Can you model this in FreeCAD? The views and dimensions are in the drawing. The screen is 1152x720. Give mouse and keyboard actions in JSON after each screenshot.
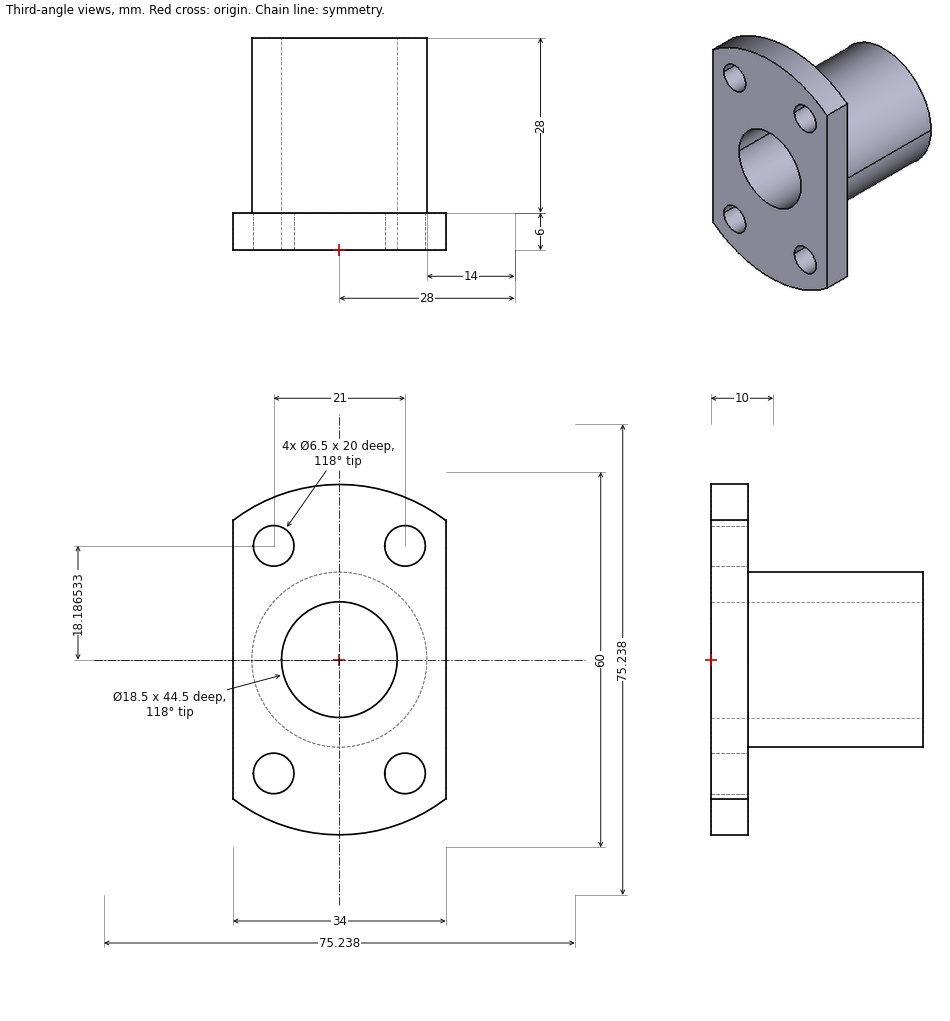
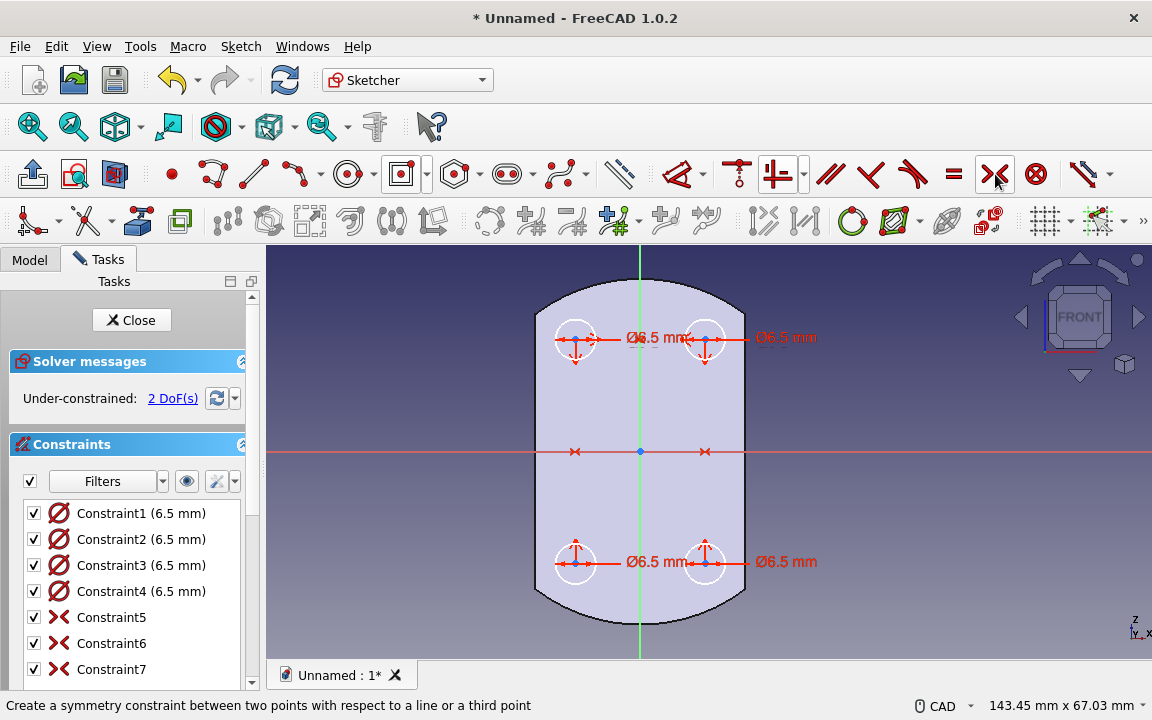
{"action": "left_click", "coordinate": [676, 174]}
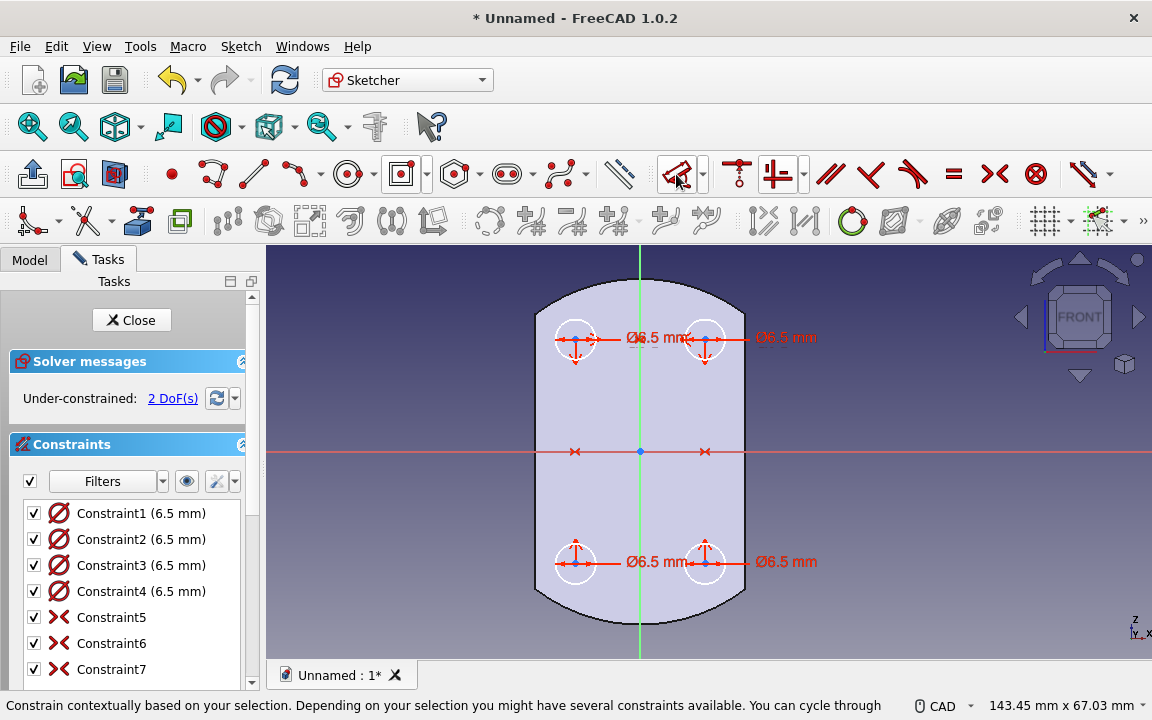
{"action": "left_click", "coordinate": [576, 340]}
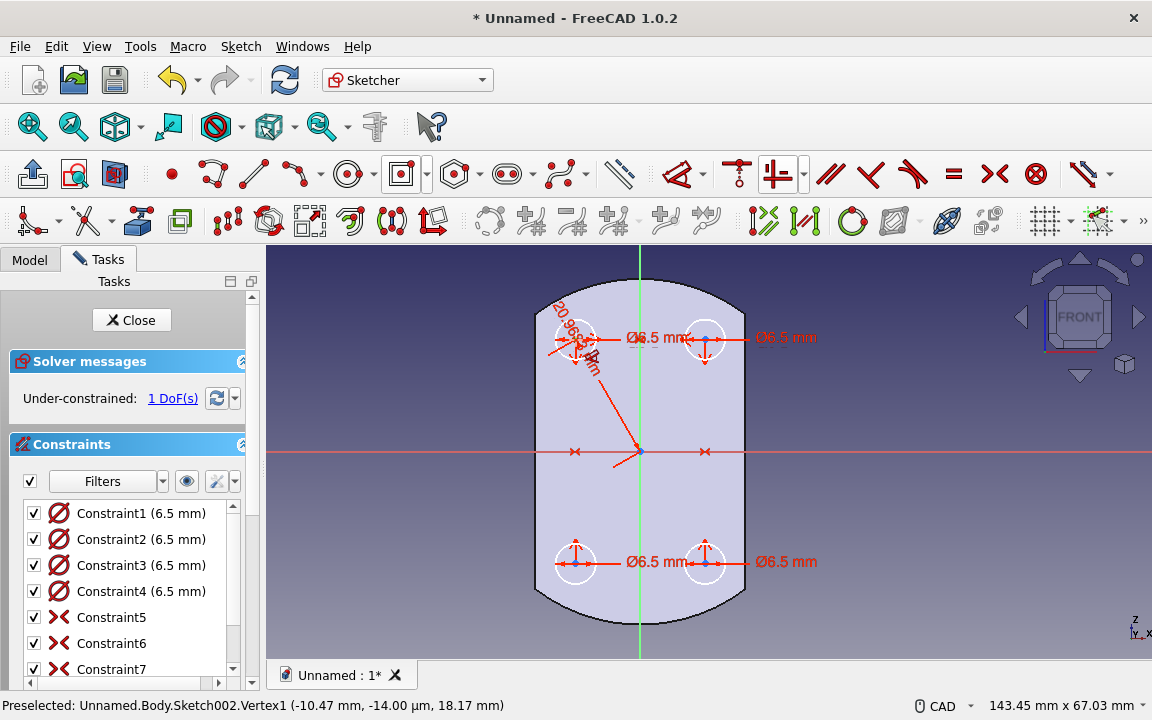
{"action": "left_click", "coordinate": [705, 340]}
{"action": "left_click", "coordinate": [611, 306]}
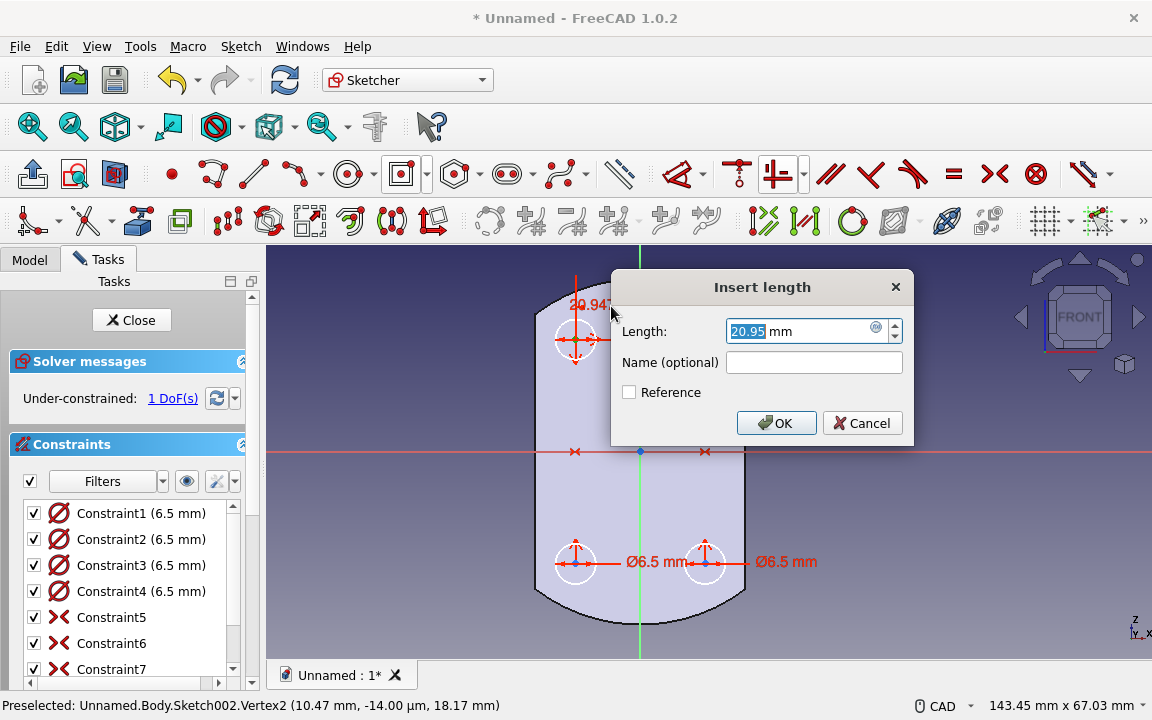
{"action": "type", "text": "21"}
{"action": "key", "text": "Return"}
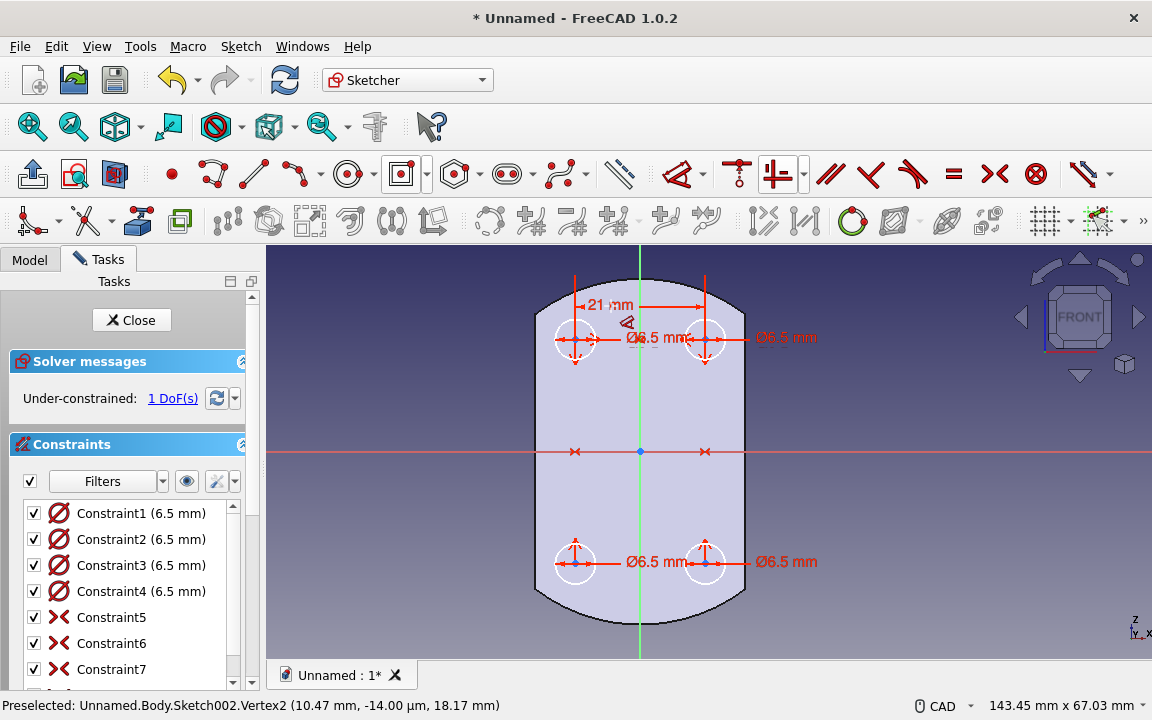
{"action": "left_click", "coordinate": [575, 340]}
{"action": "left_click", "coordinate": [541, 396]}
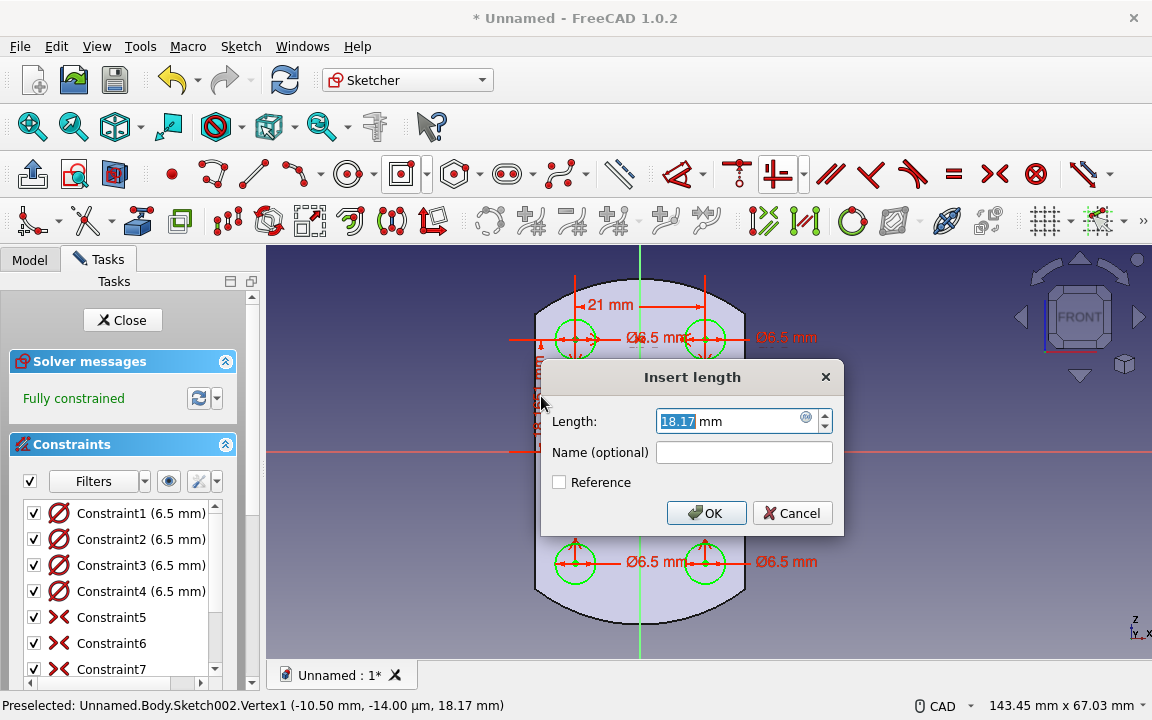
{"action": "type", "text": "18.186533"}
{"action": "key", "text": "Return"}
{"action": "key", "text": "Escape"}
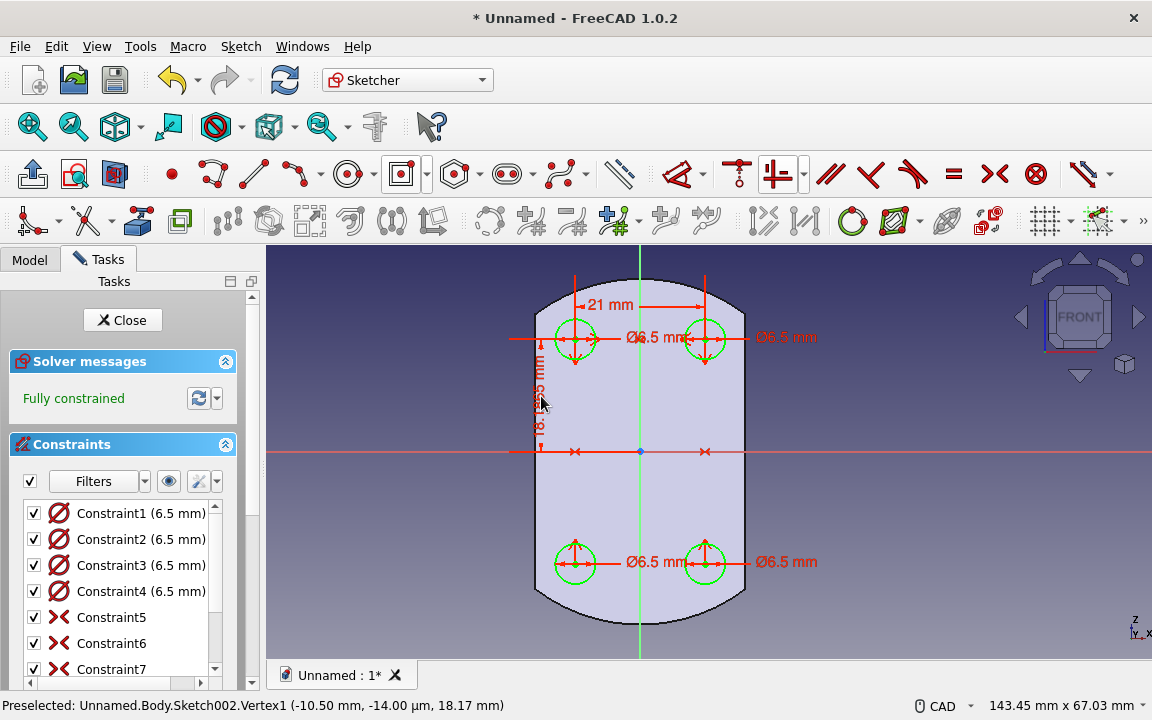
{"action": "left_click", "coordinate": [123, 320]}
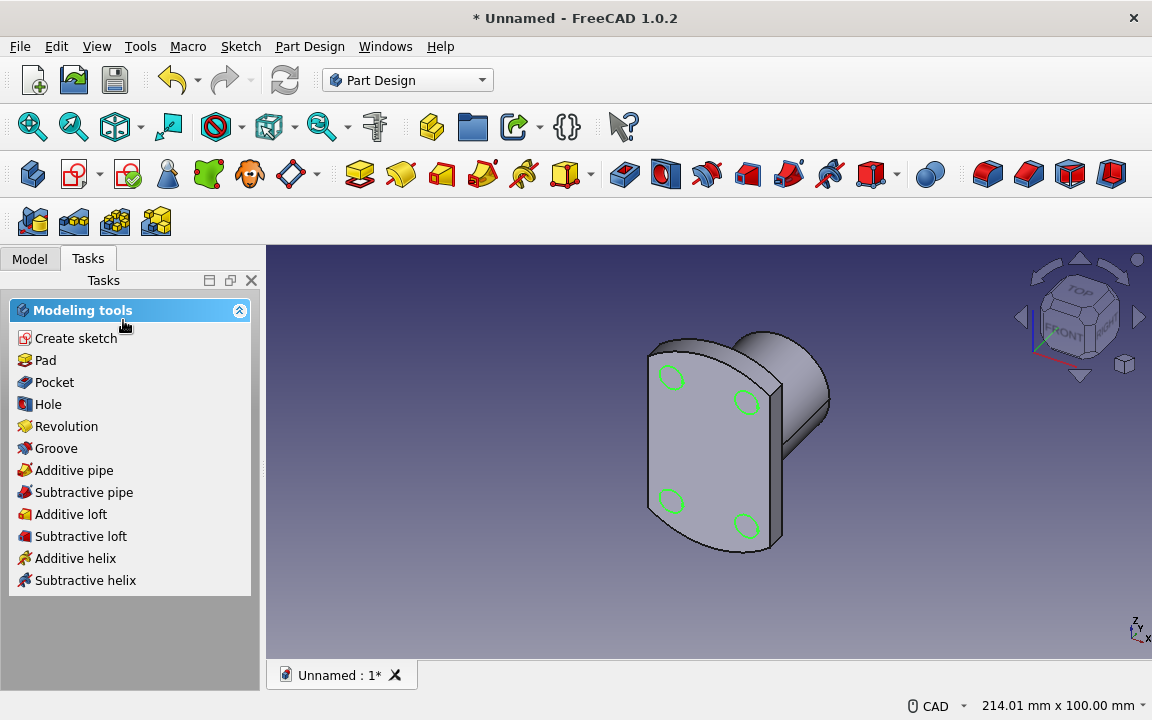
{"action": "left_click", "coordinate": [666, 174]}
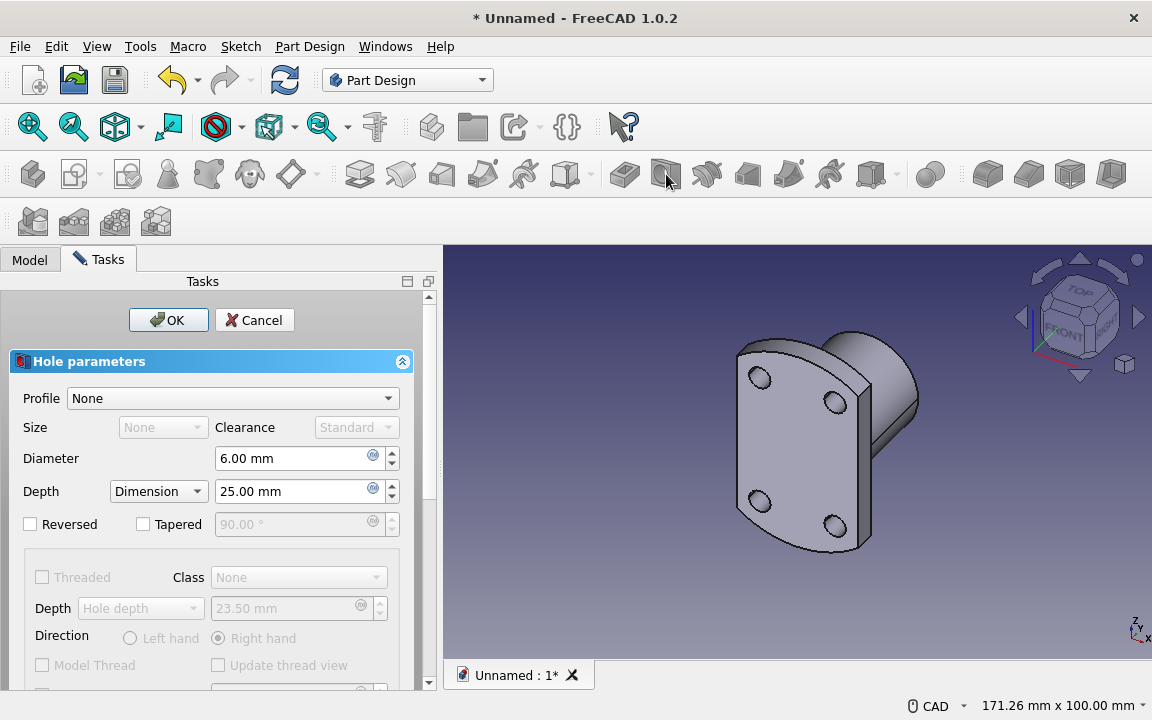
{"action": "triple_click", "coordinate": [300, 458]}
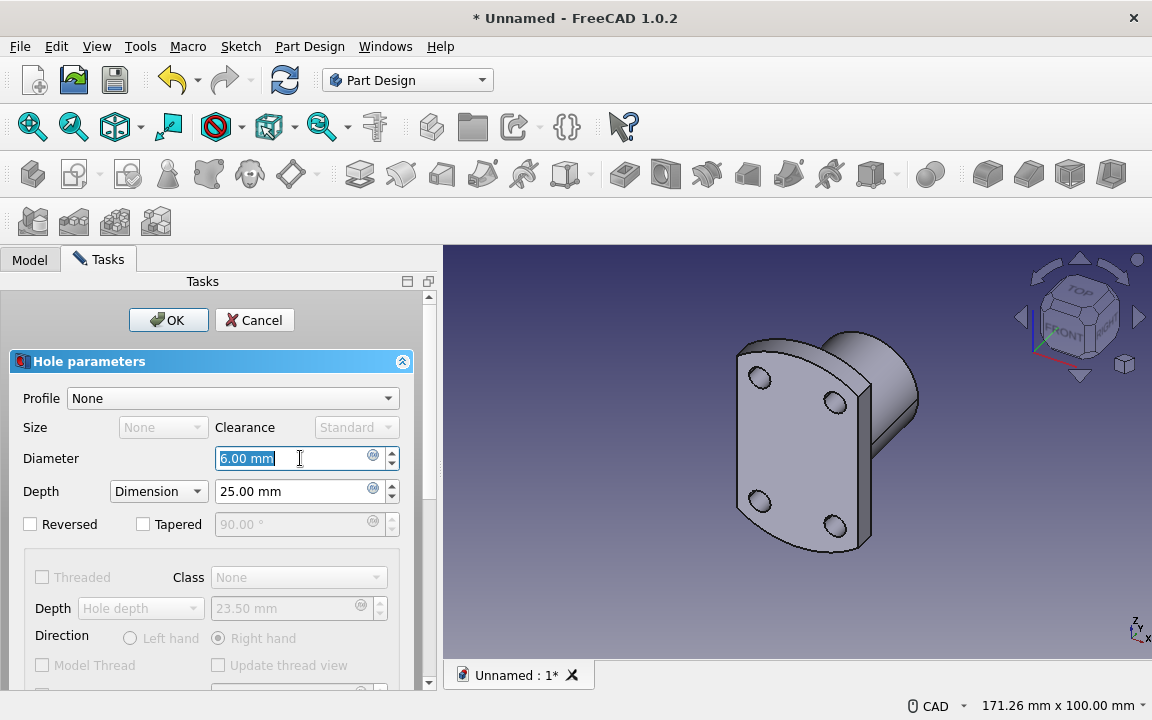
{"action": "type", "text": "6.5"}
{"action": "key", "text": "Tab"}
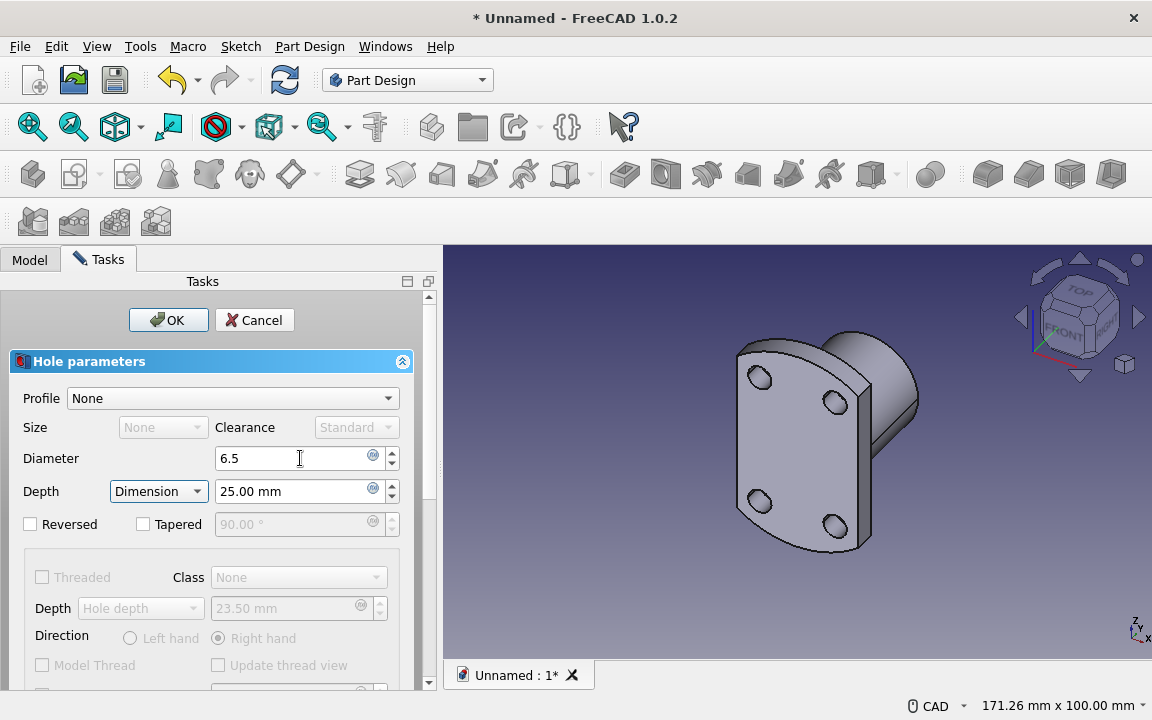
{"action": "triple_click", "coordinate": [300, 492]}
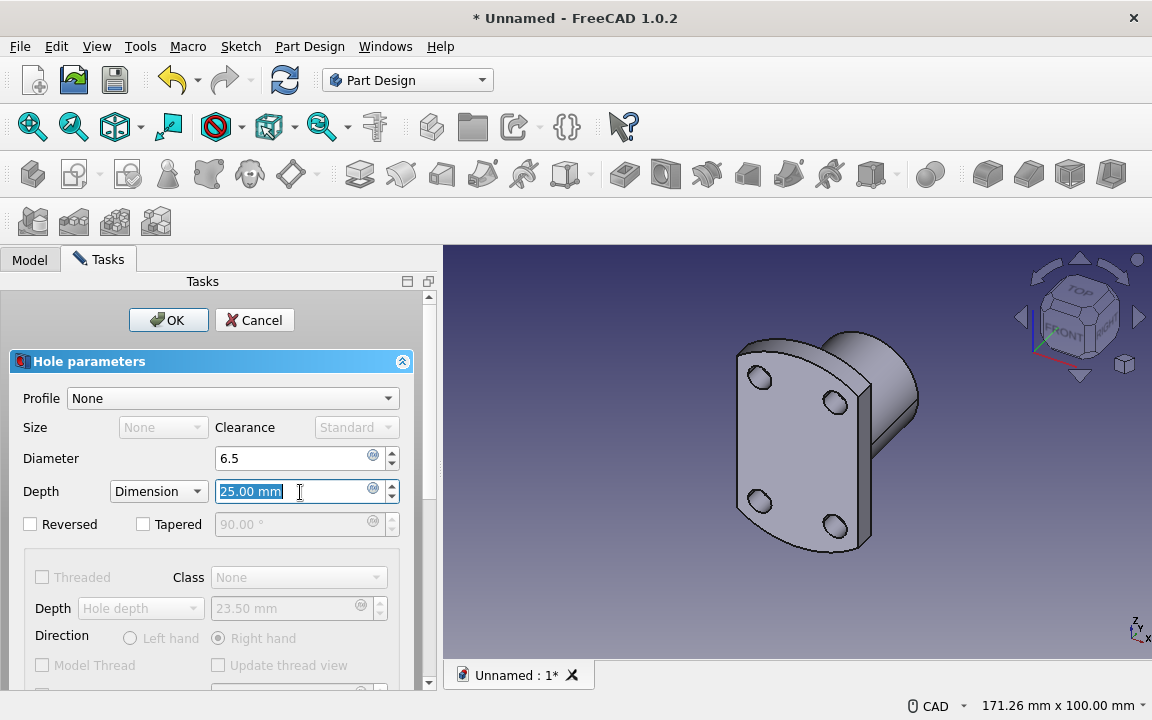
{"action": "type", "text": "20"}
{"action": "key", "text": "Tab"}